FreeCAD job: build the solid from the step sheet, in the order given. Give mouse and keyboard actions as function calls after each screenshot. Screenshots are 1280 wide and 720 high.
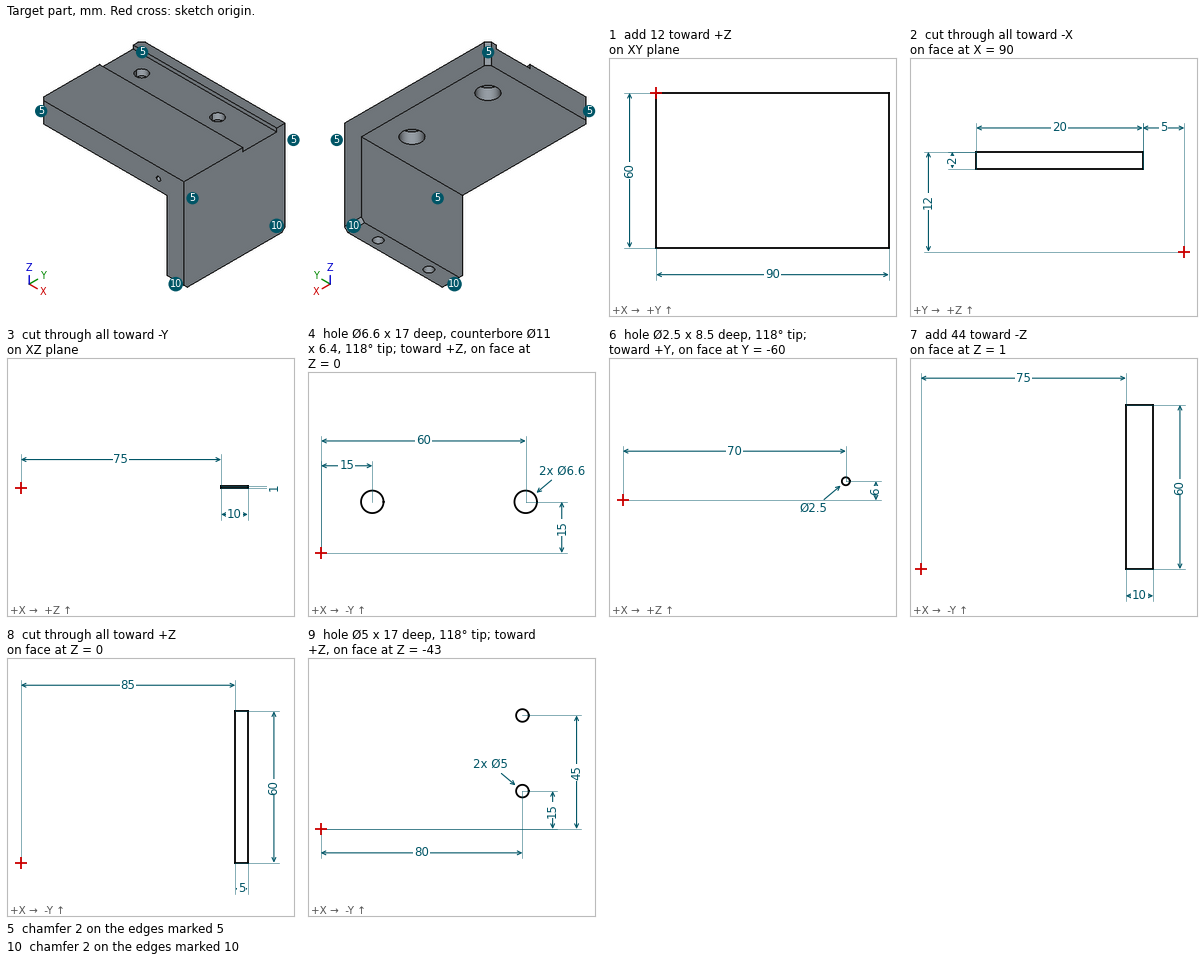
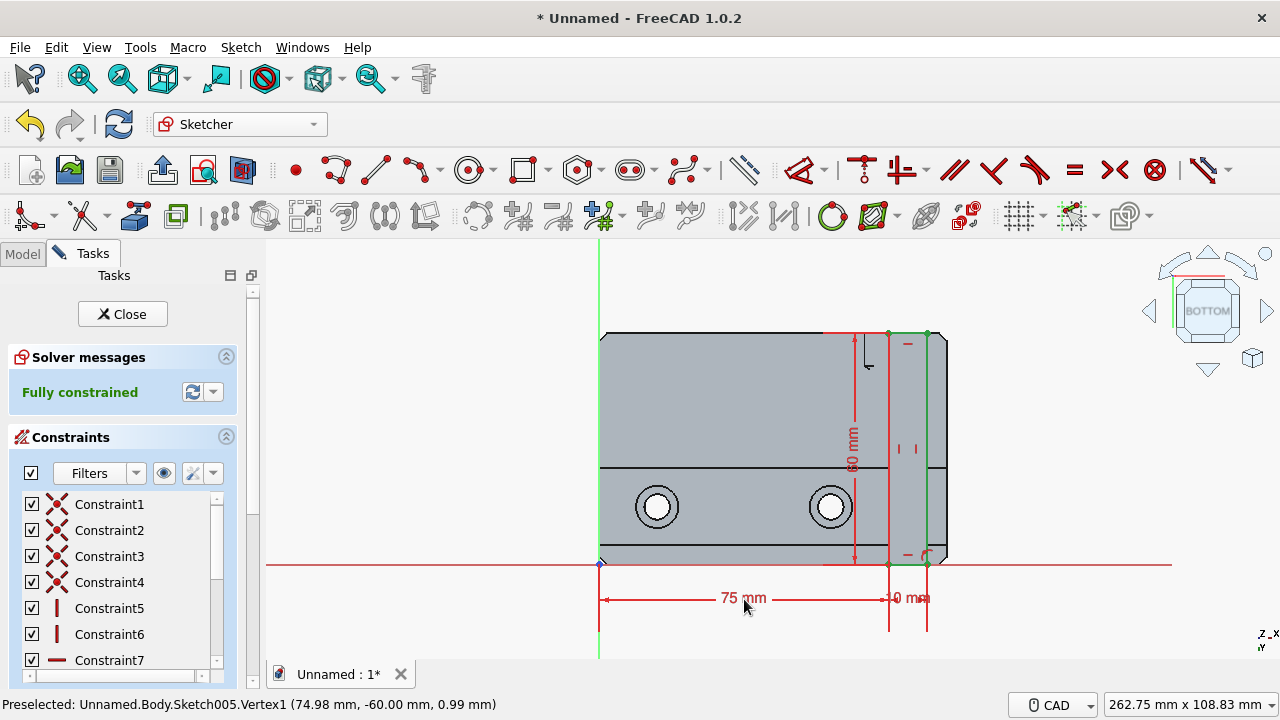
click(123, 314)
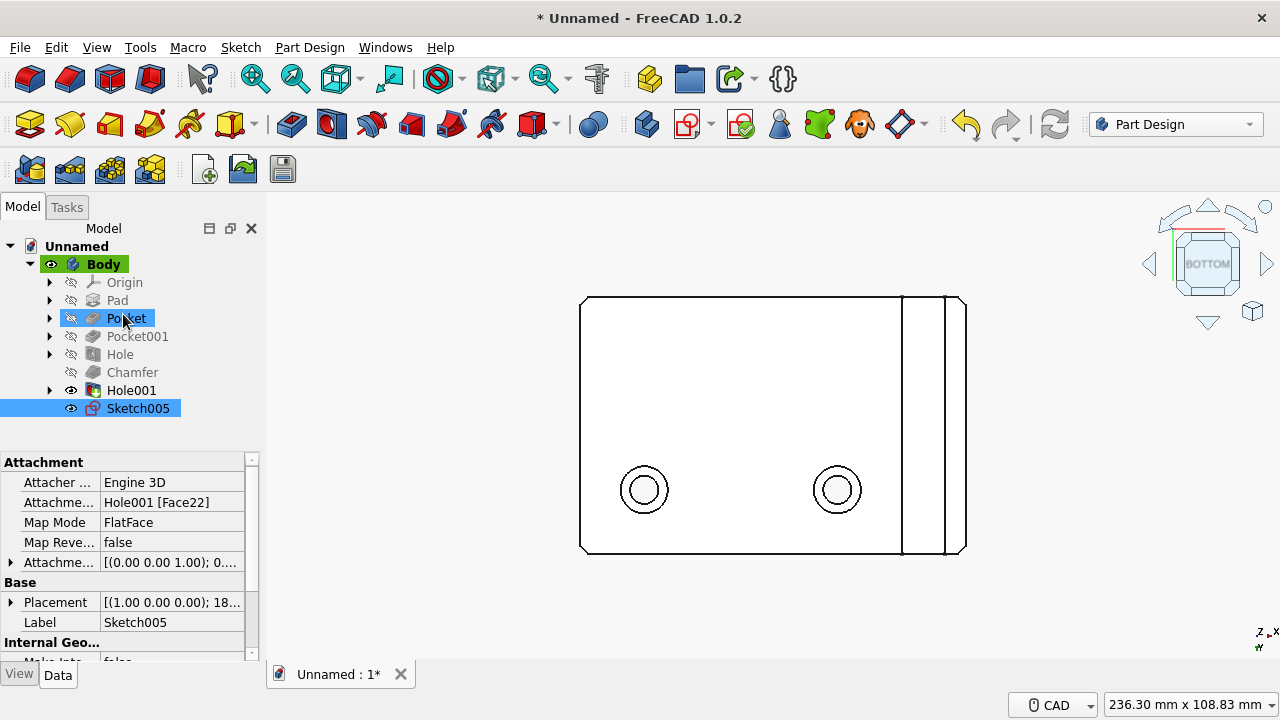
click(30, 124)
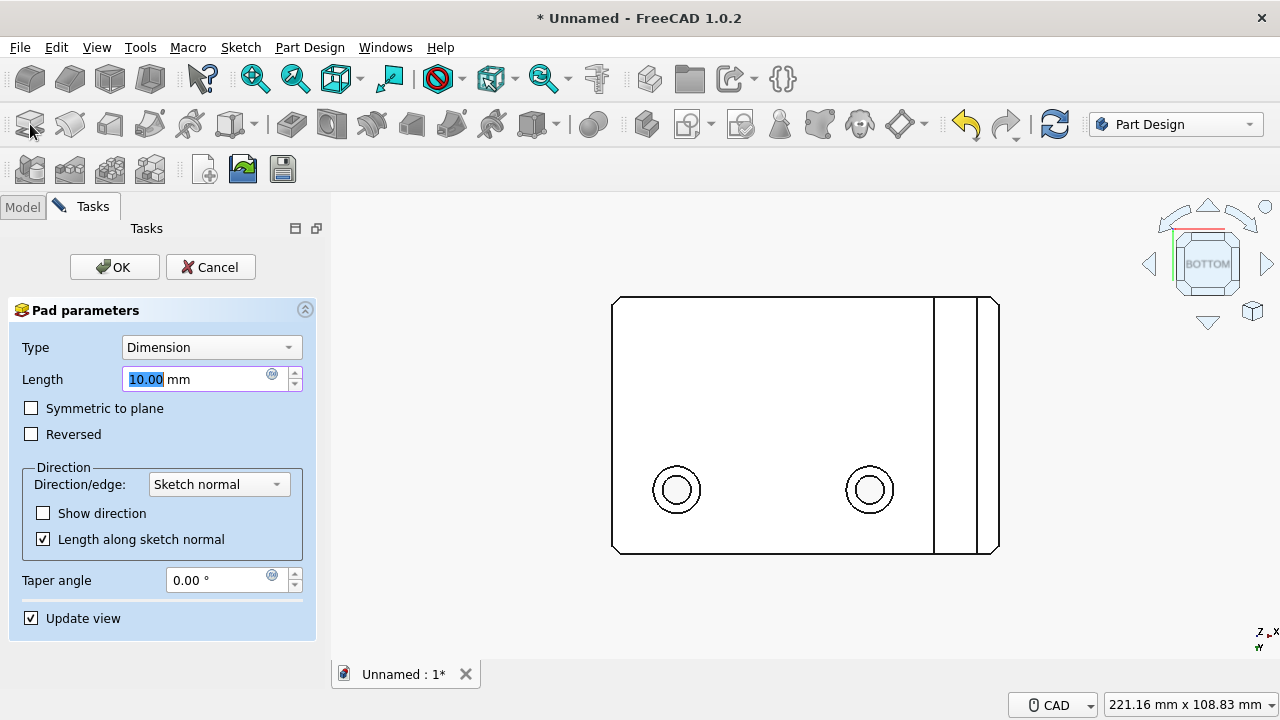
text(44)
key(Tab)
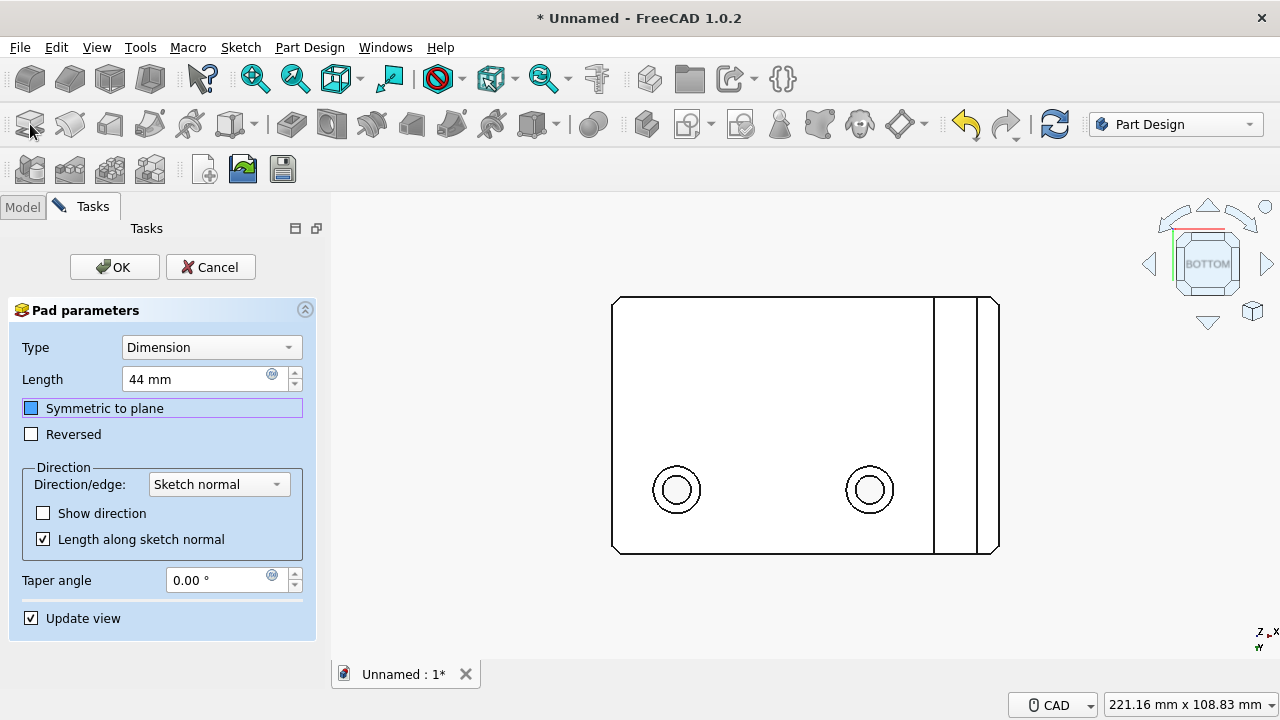
click(115, 267)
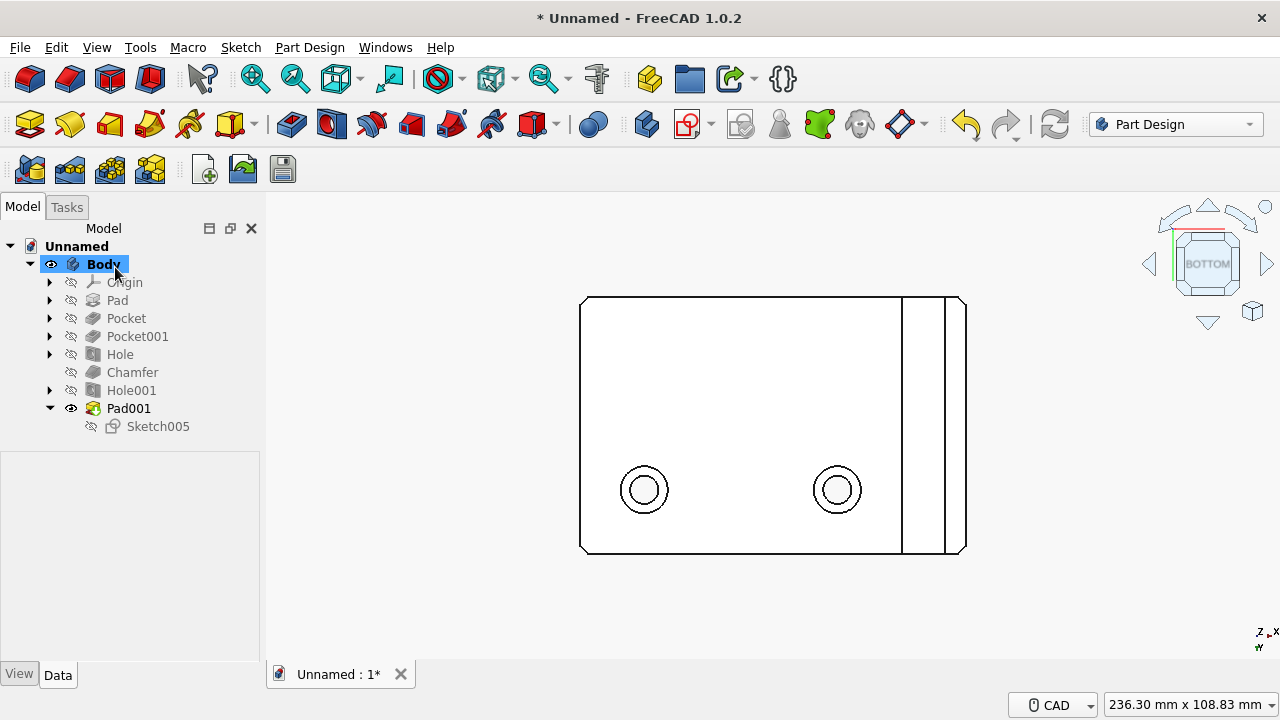
click(741, 425)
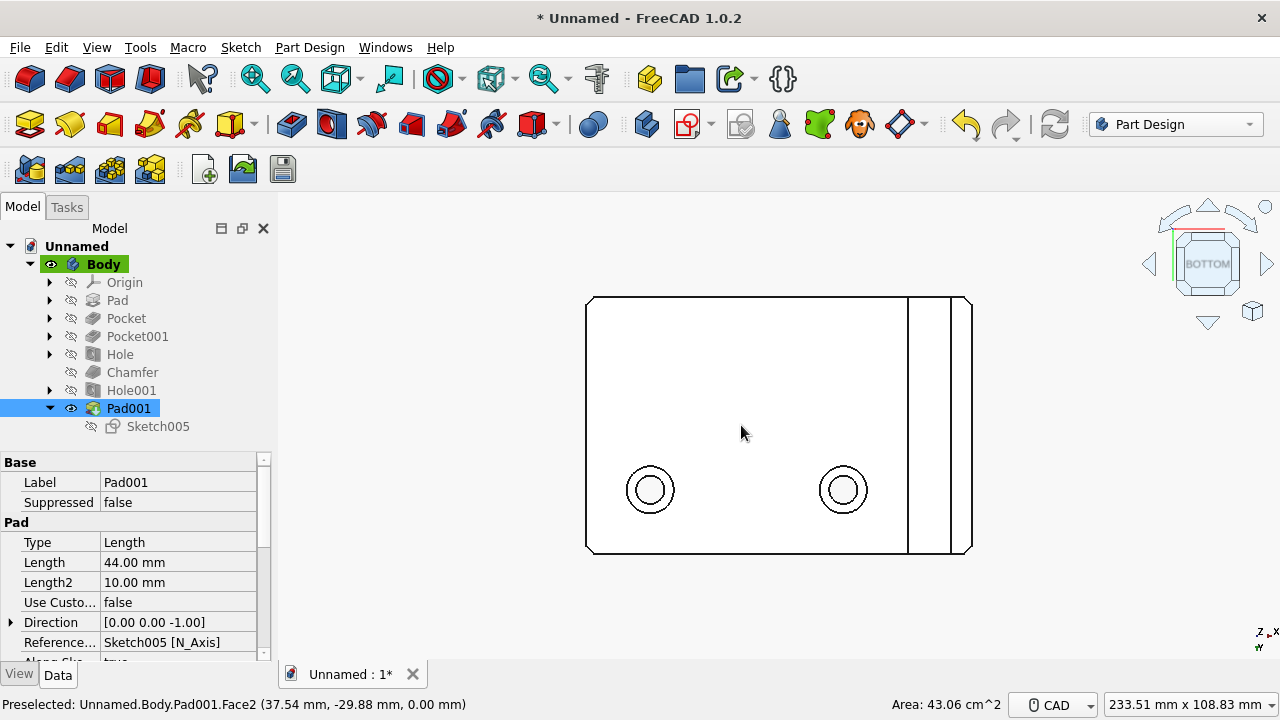
click(688, 124)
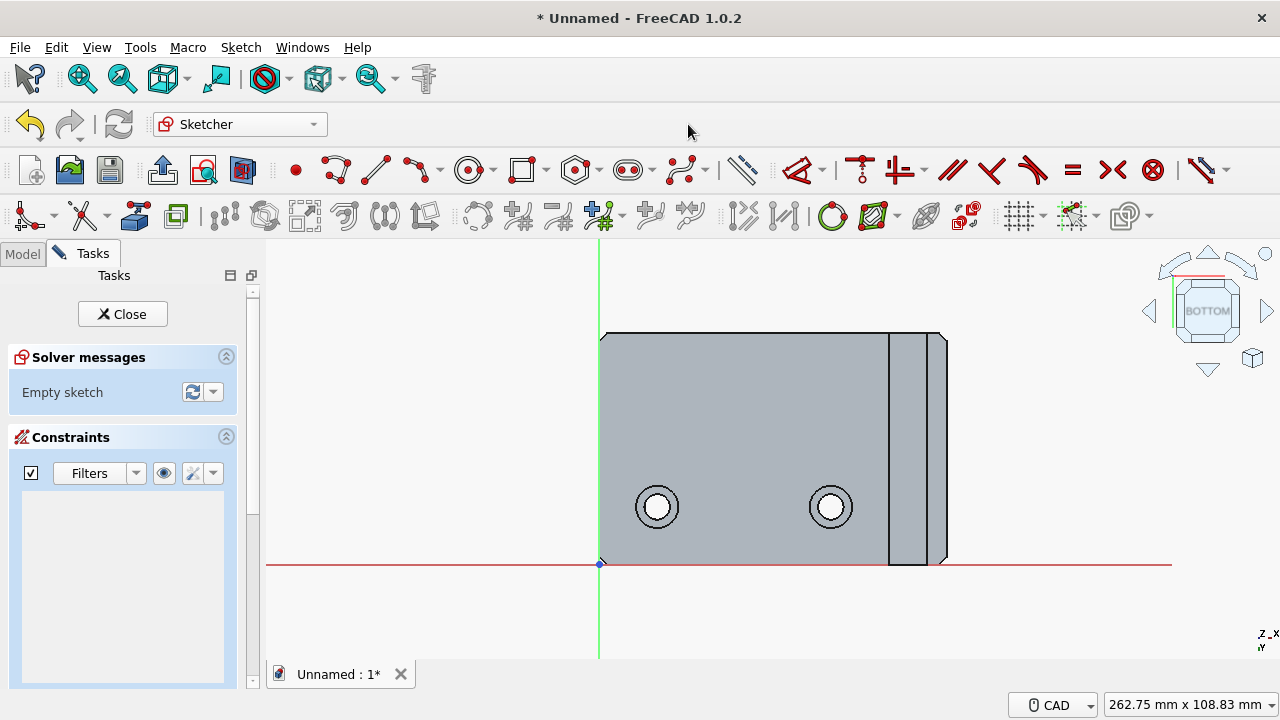
click(244, 170)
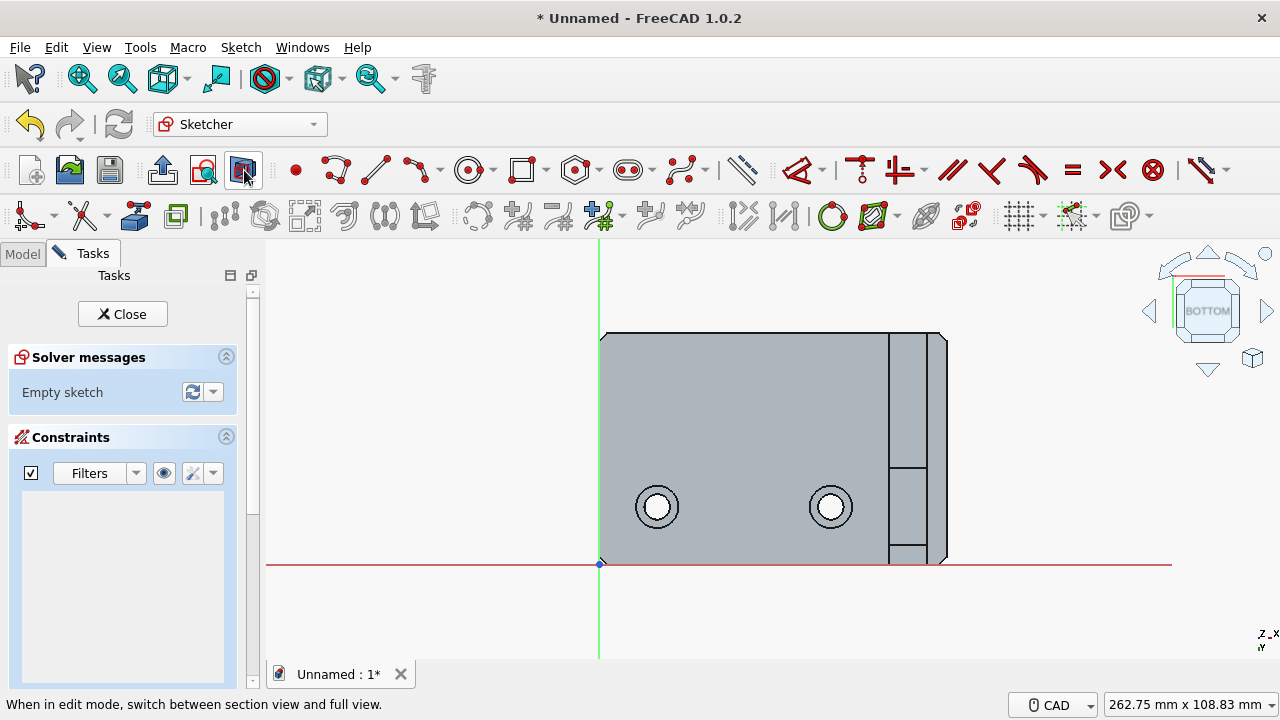
click(522, 170)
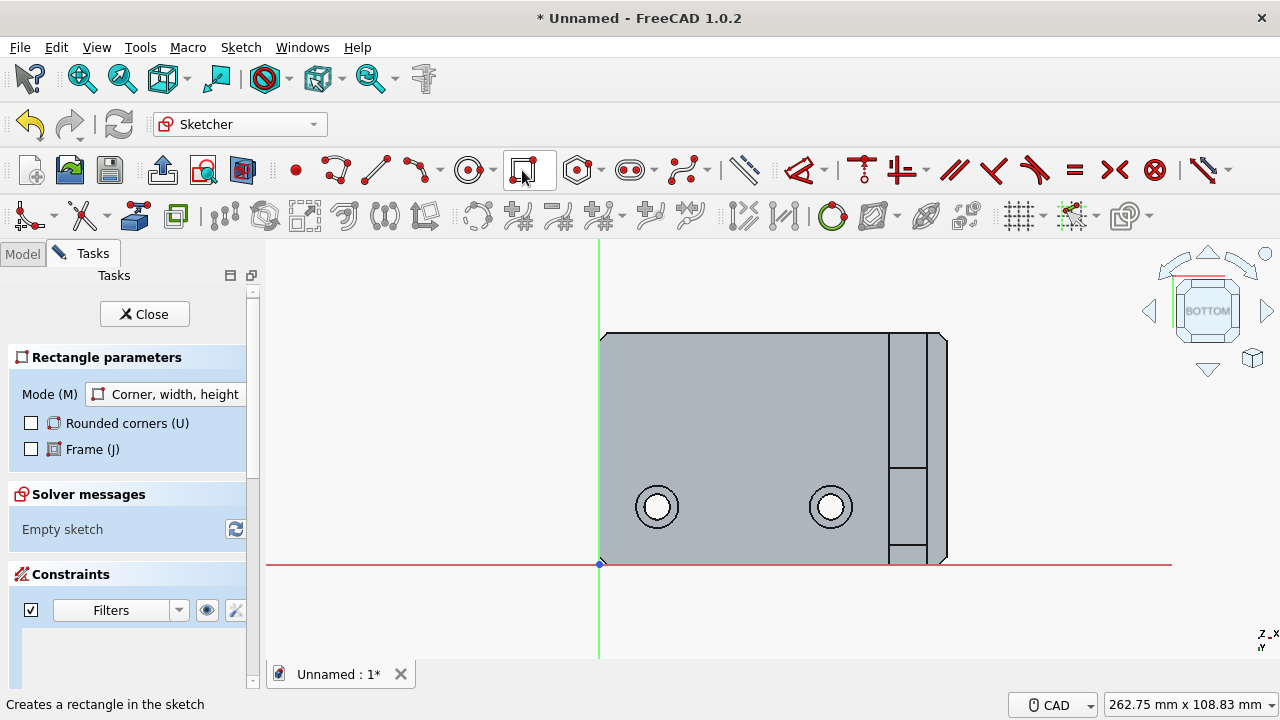
click(927, 333)
click(947, 565)
key(Escape)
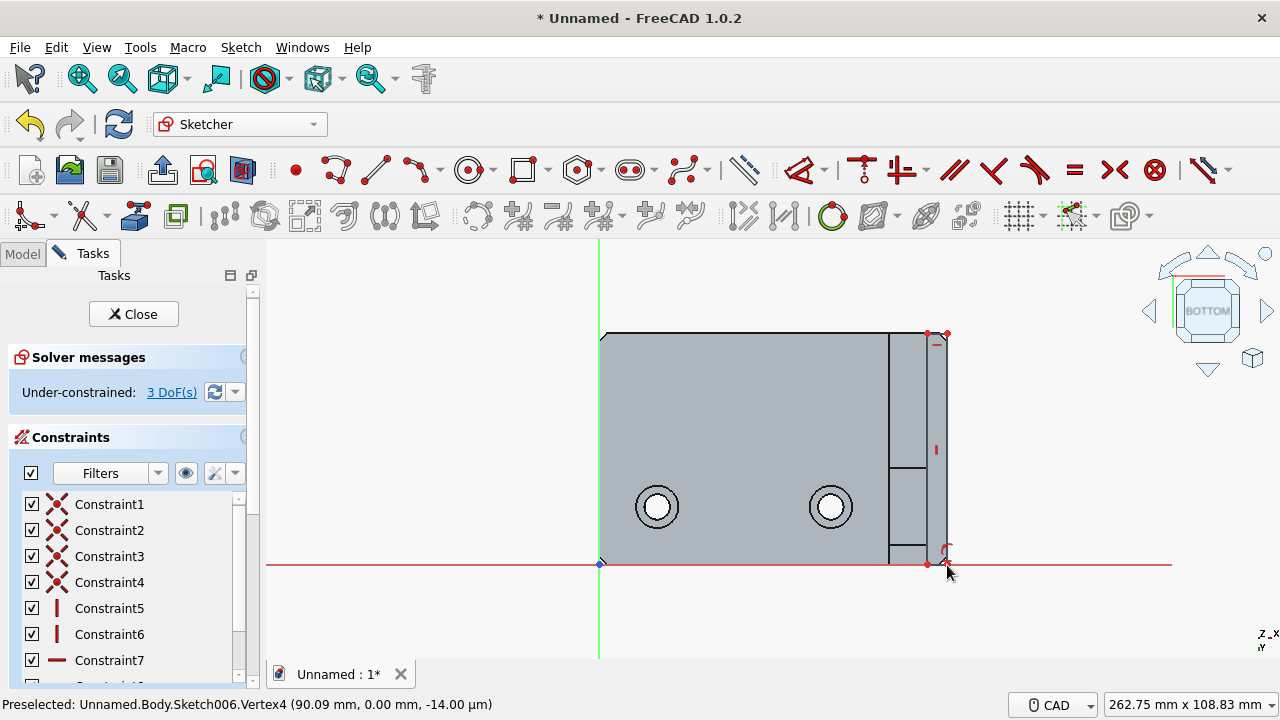
click(800, 170)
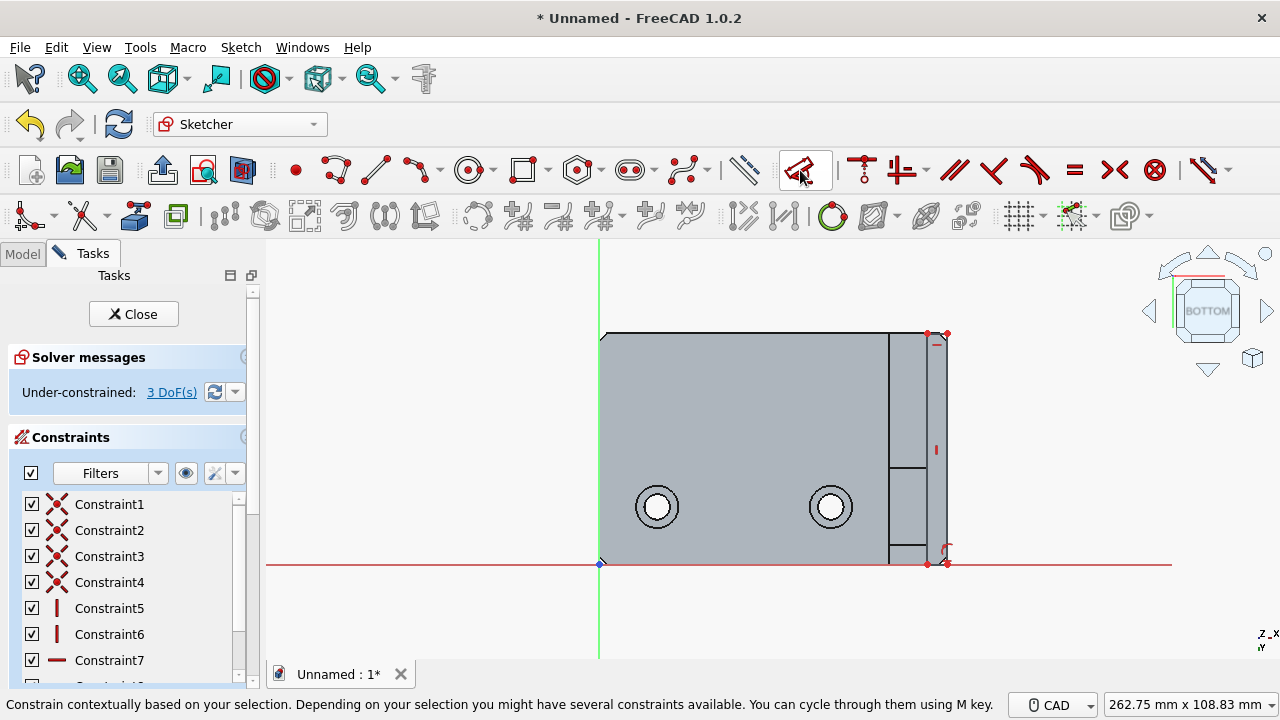
scroll(937, 565, up, 4)